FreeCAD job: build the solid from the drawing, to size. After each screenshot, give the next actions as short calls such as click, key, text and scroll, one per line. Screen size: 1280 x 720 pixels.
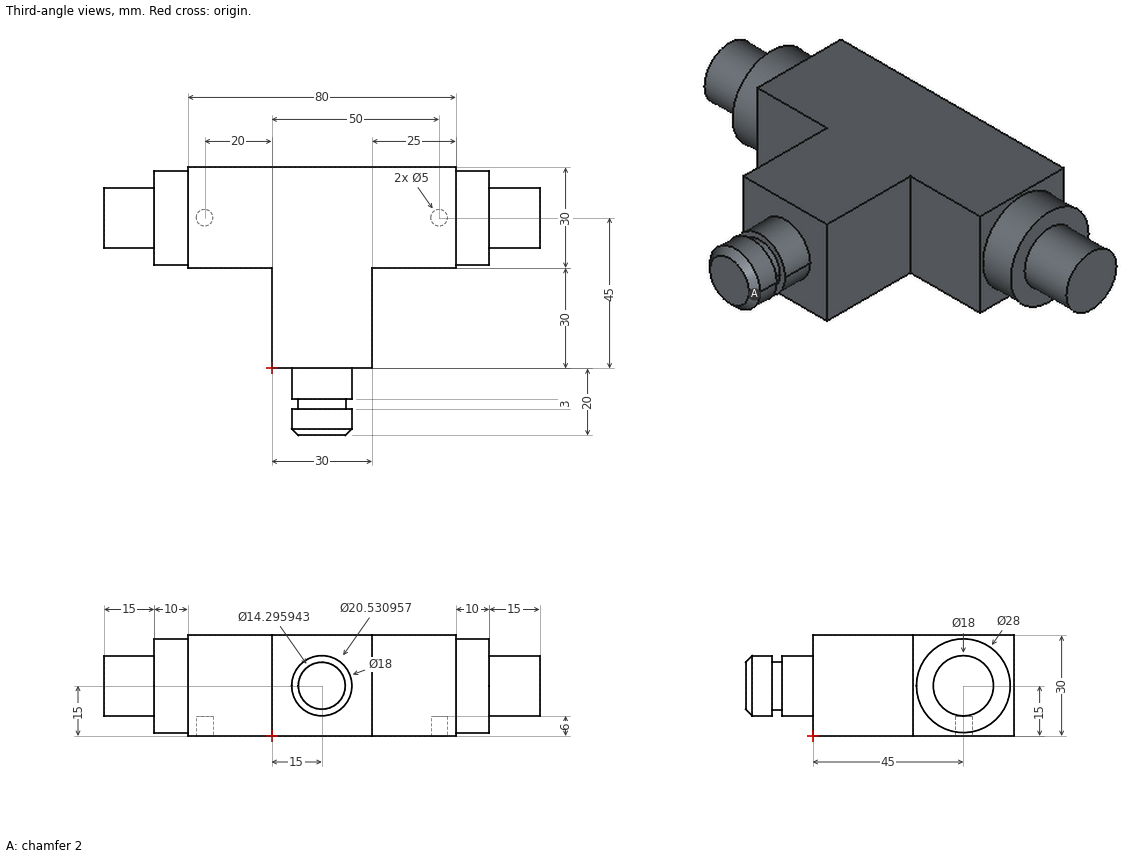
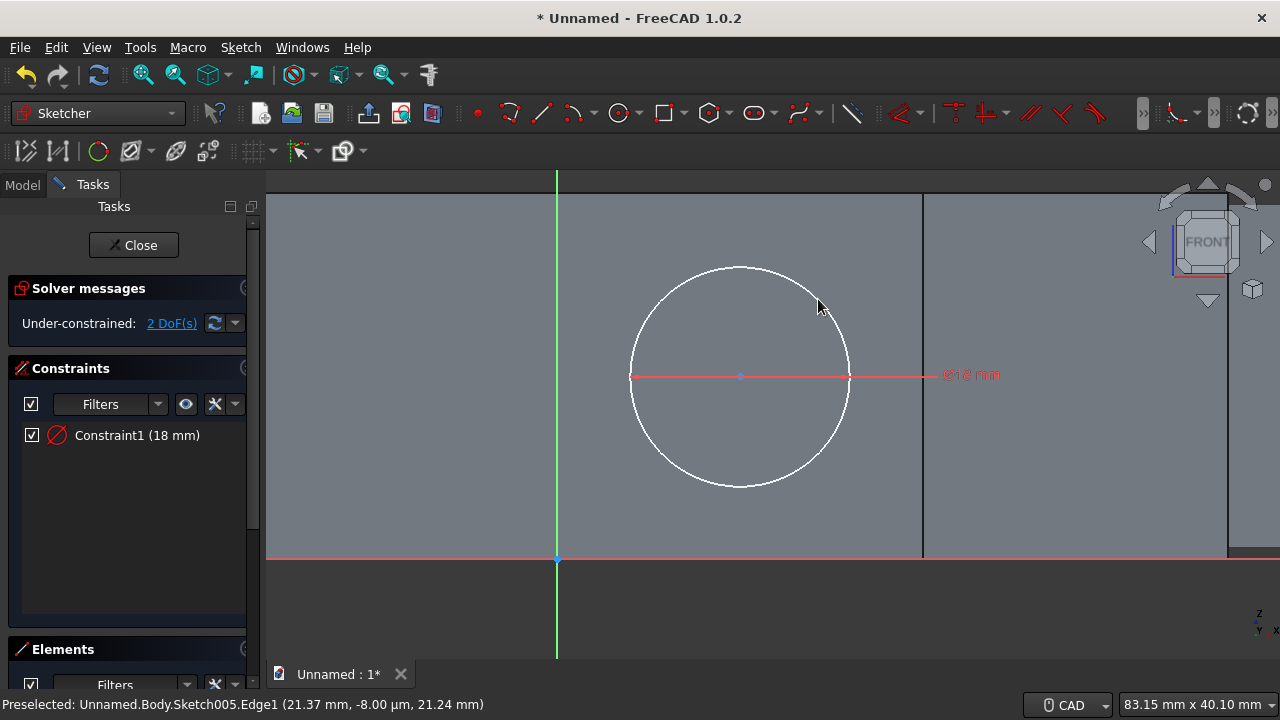
key(d)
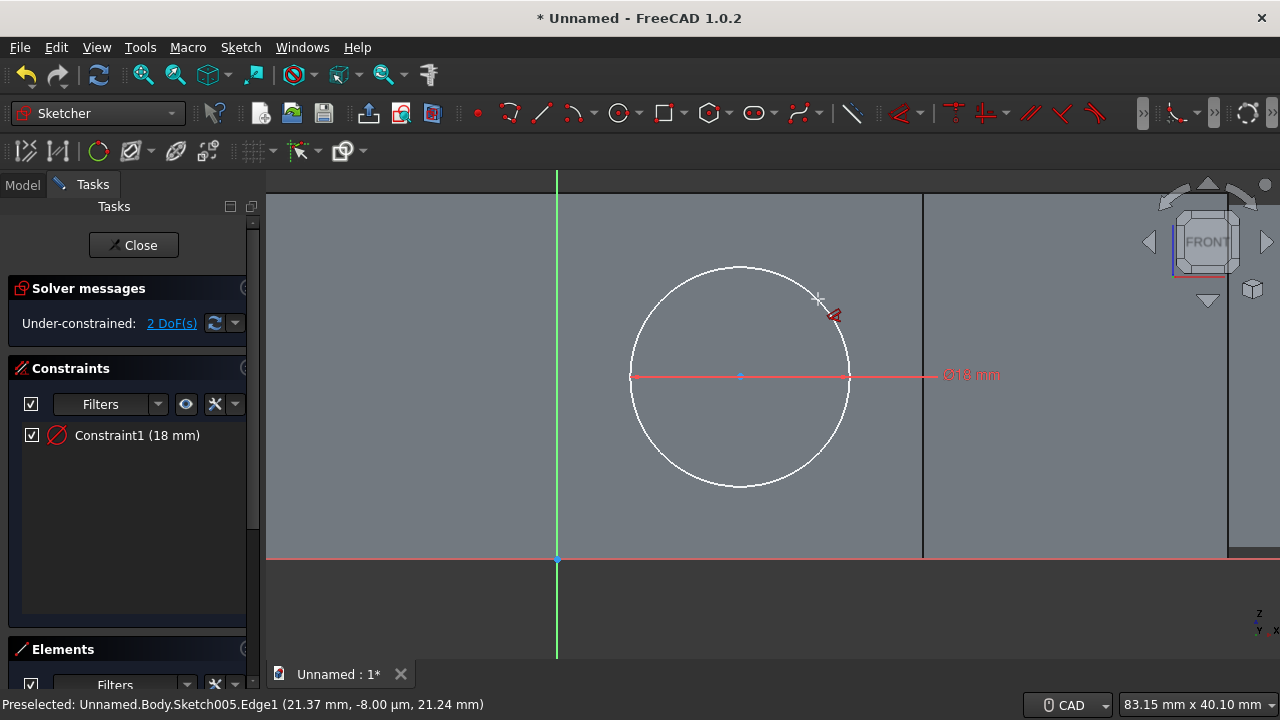
click(740, 377)
click(649, 593)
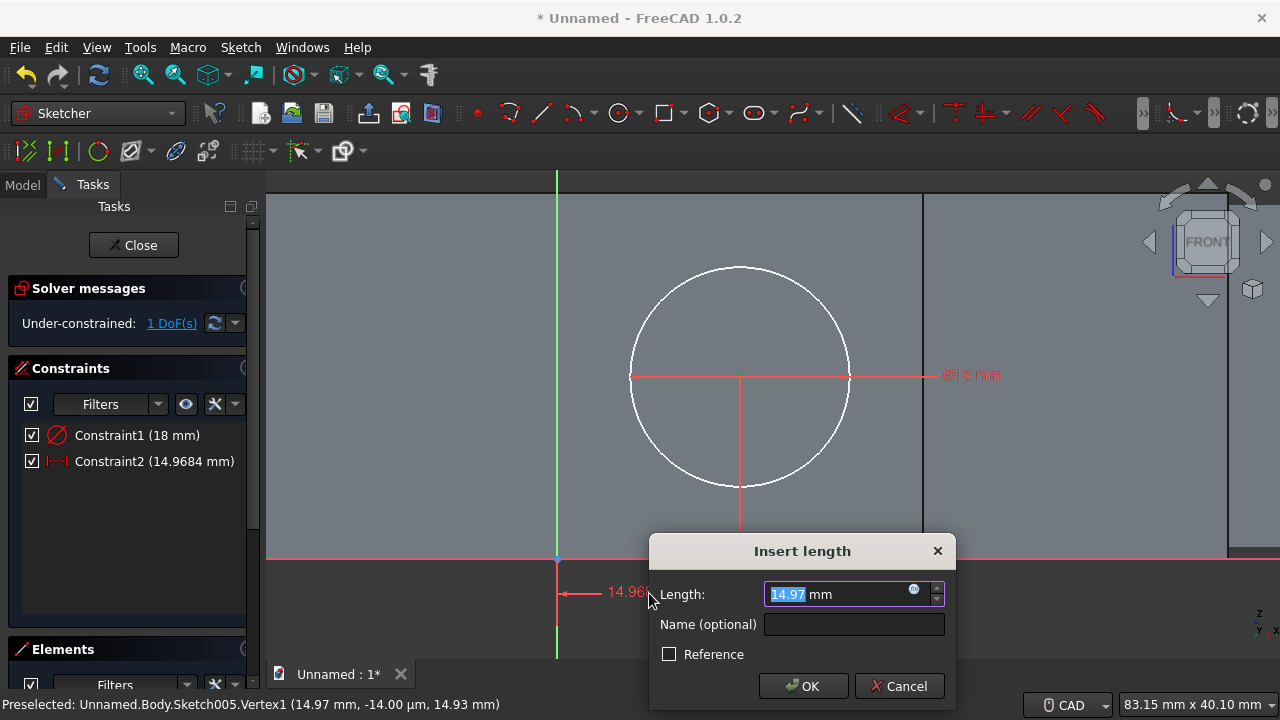
text(15)
key(Return)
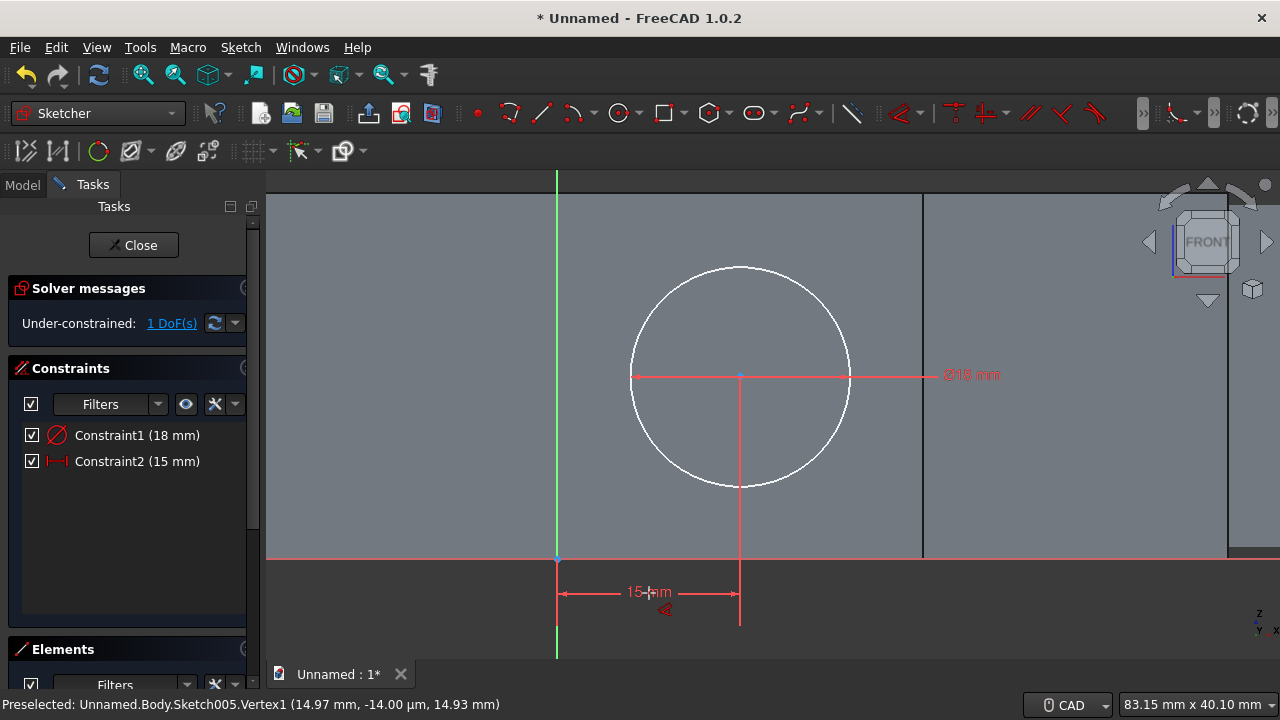
click(740, 377)
click(523, 468)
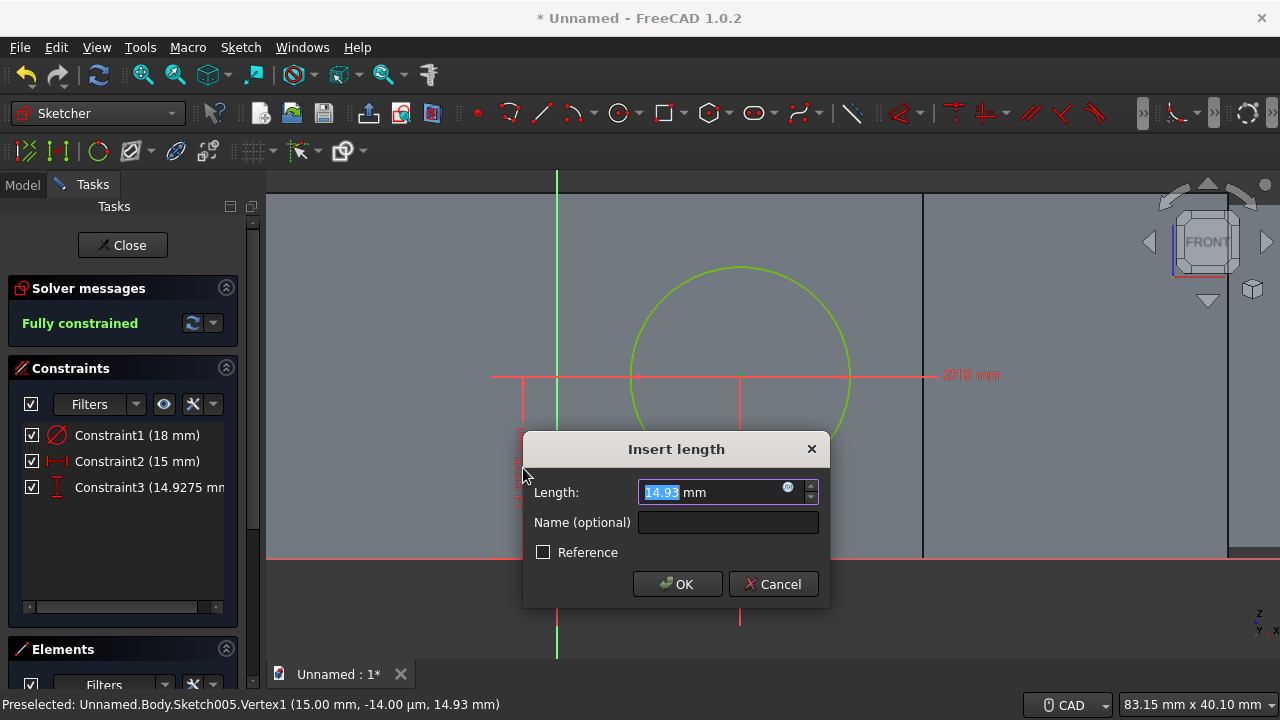
text(15)
key(Return)
key(Escape)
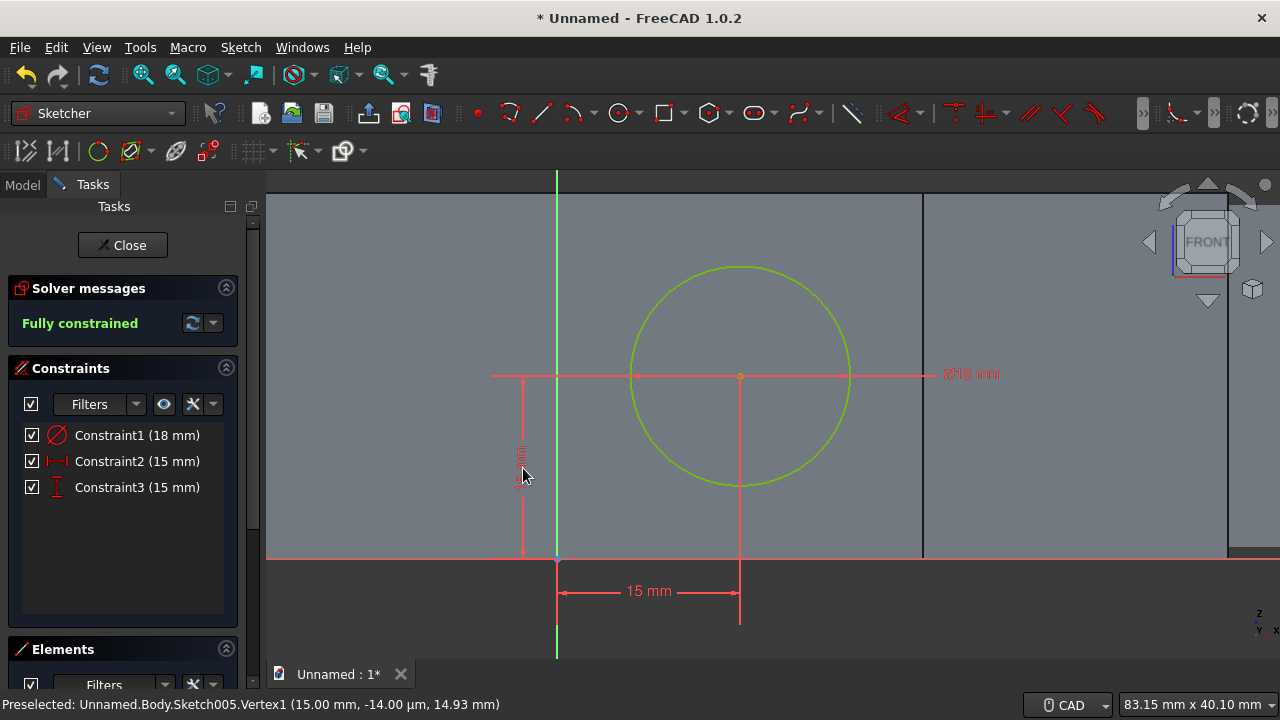
click(123, 245)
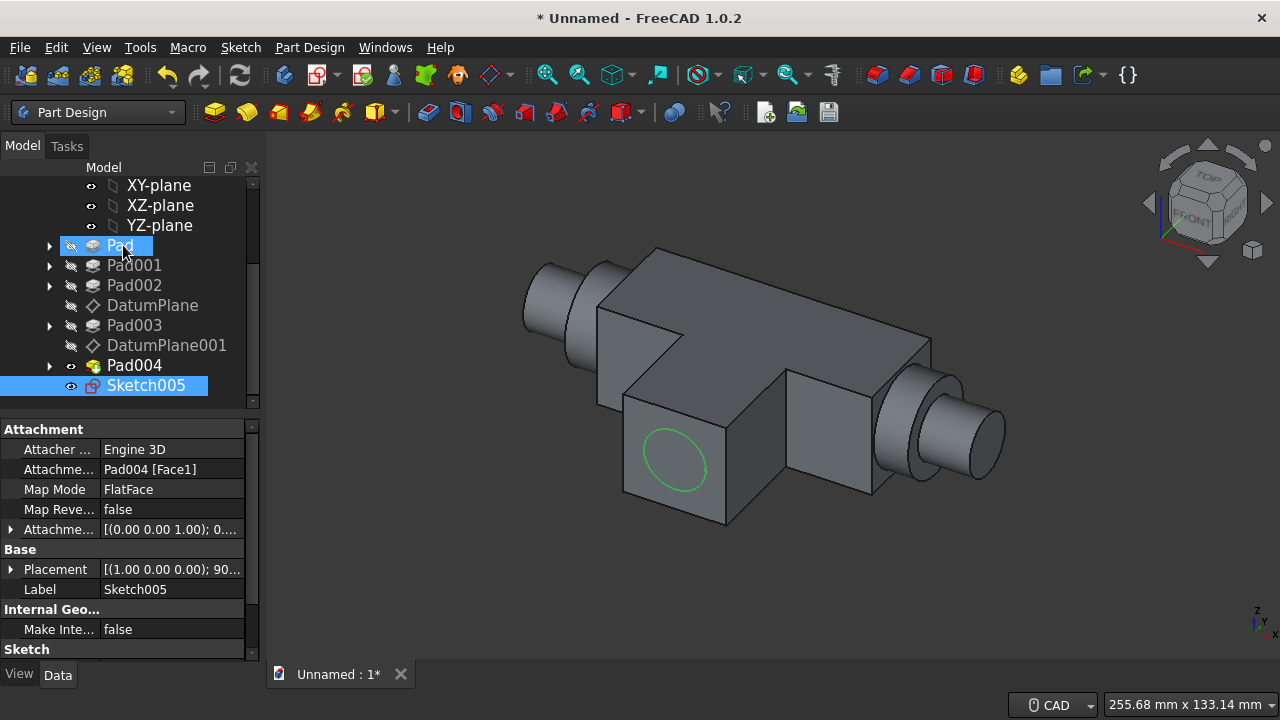
click(216, 112)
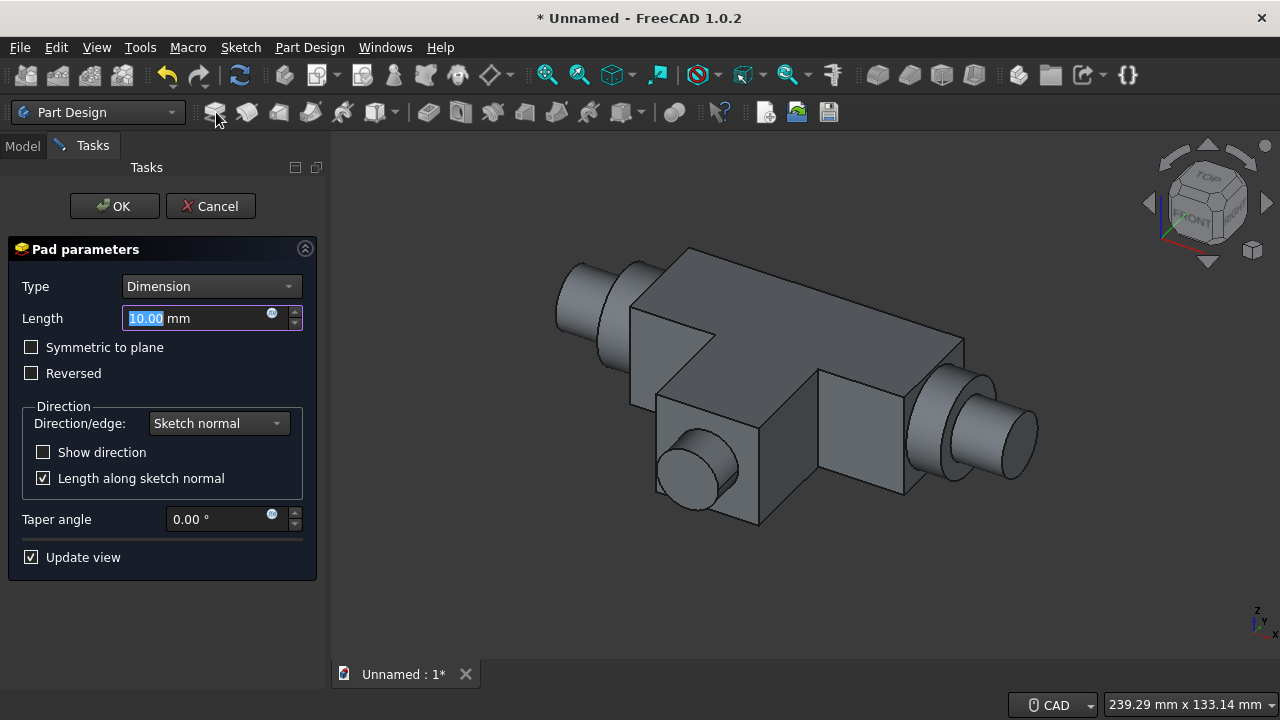
text(20)
key(Tab)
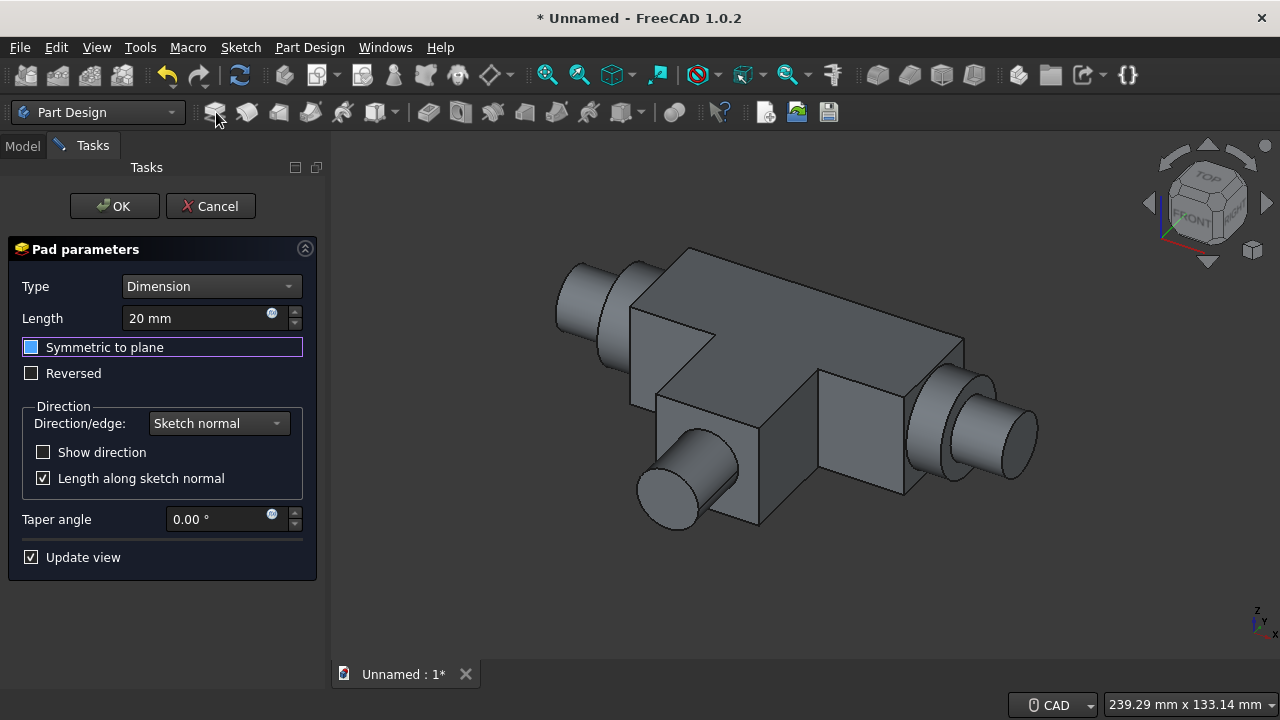
click(115, 206)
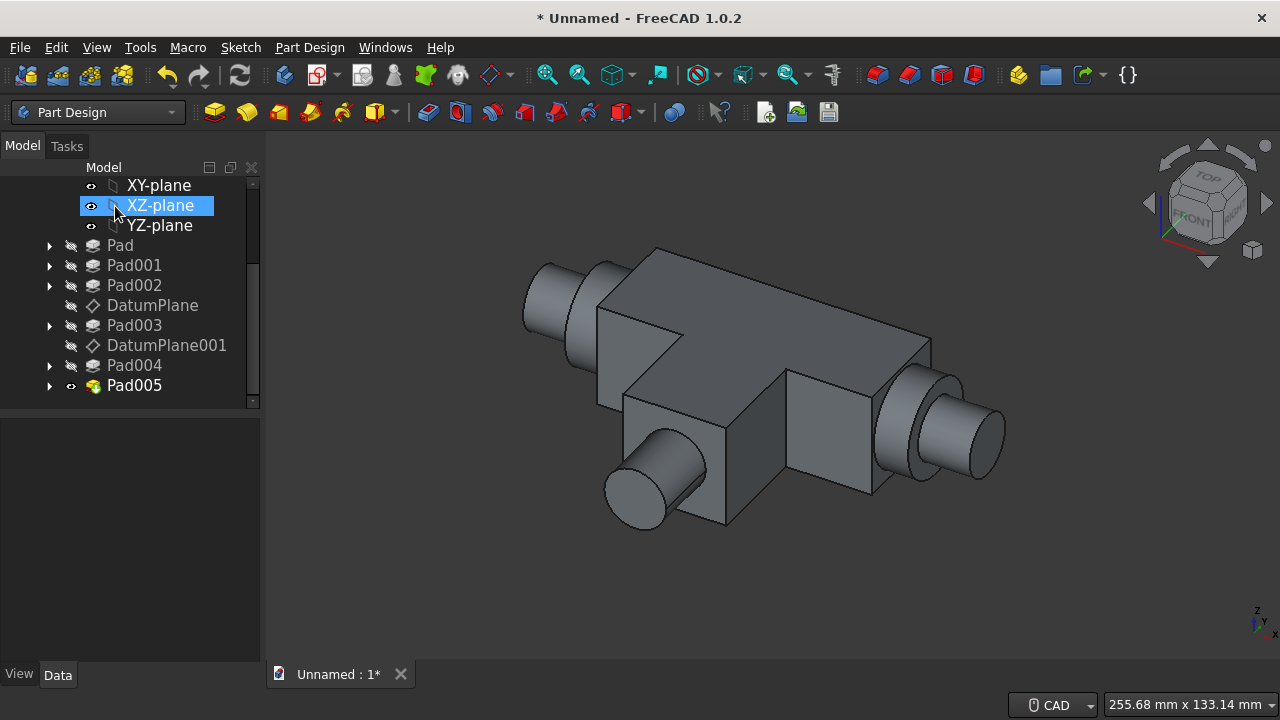
scroll(160, 281, down, 3)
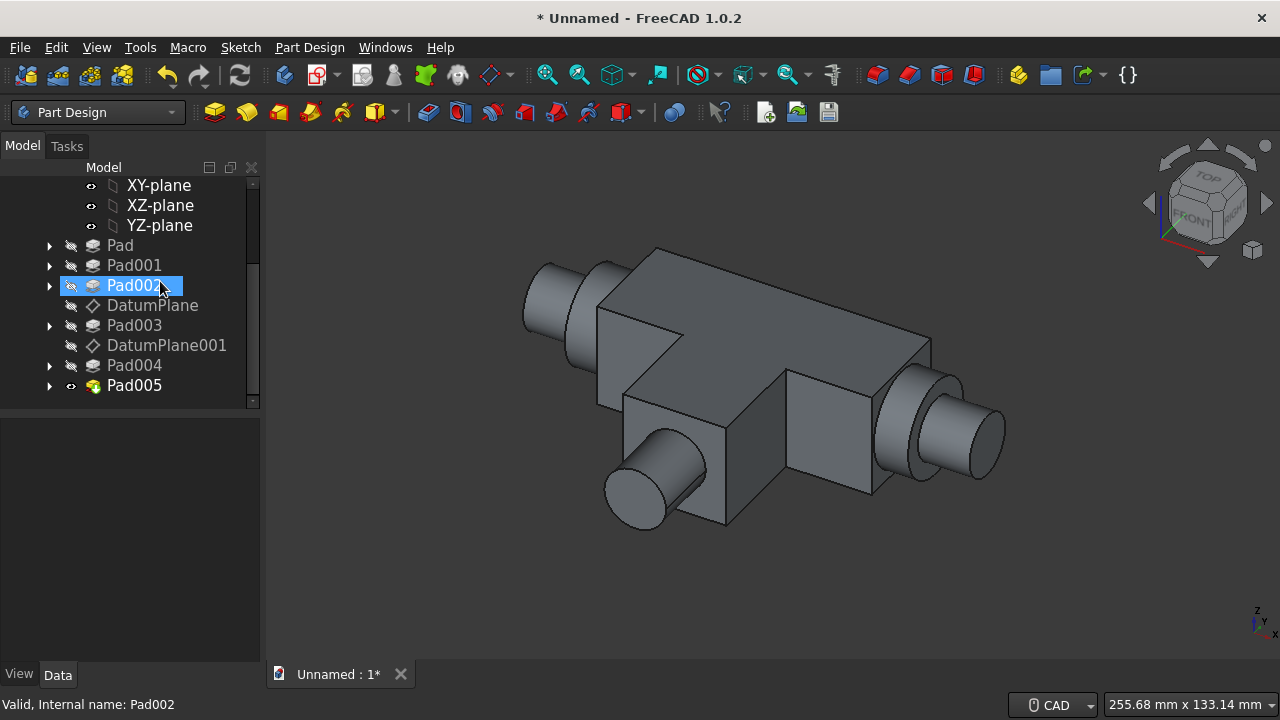
scroll(160, 281, up, 15)